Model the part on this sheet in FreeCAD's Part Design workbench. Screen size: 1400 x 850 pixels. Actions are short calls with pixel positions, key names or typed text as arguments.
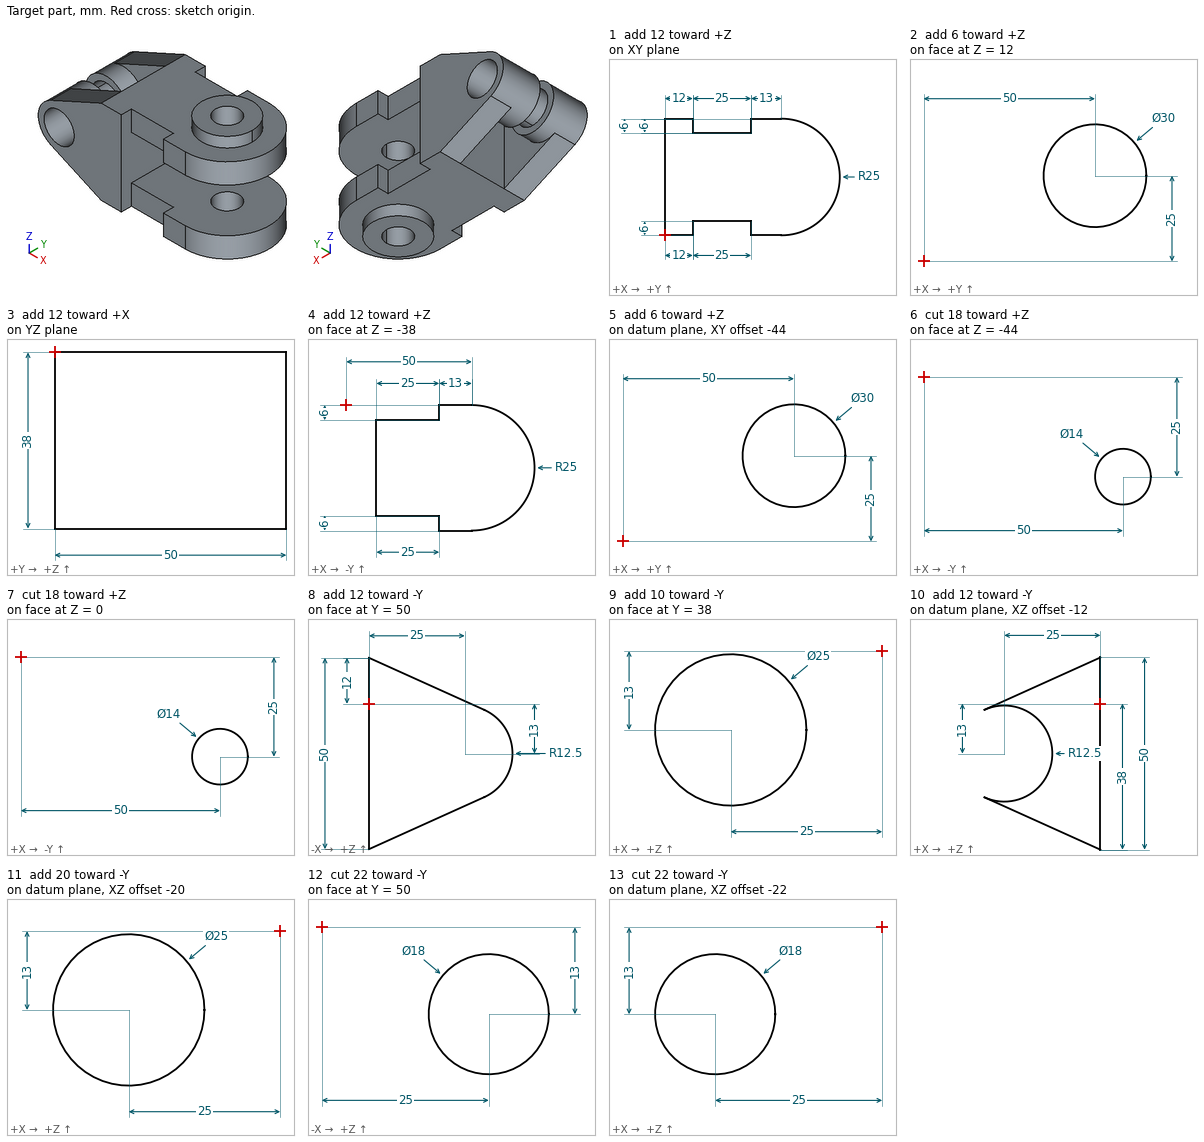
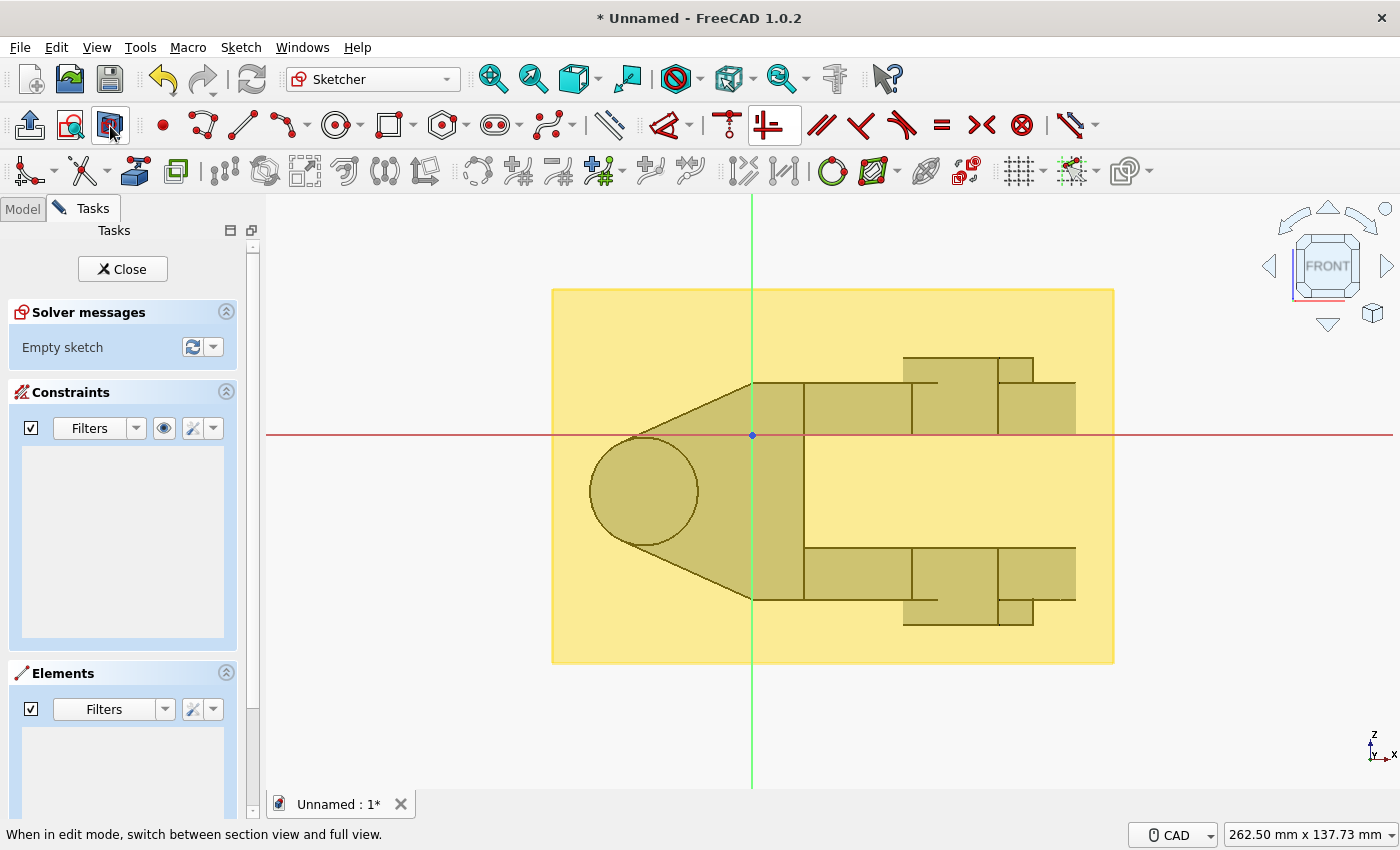
scroll(592, 491, up, 3)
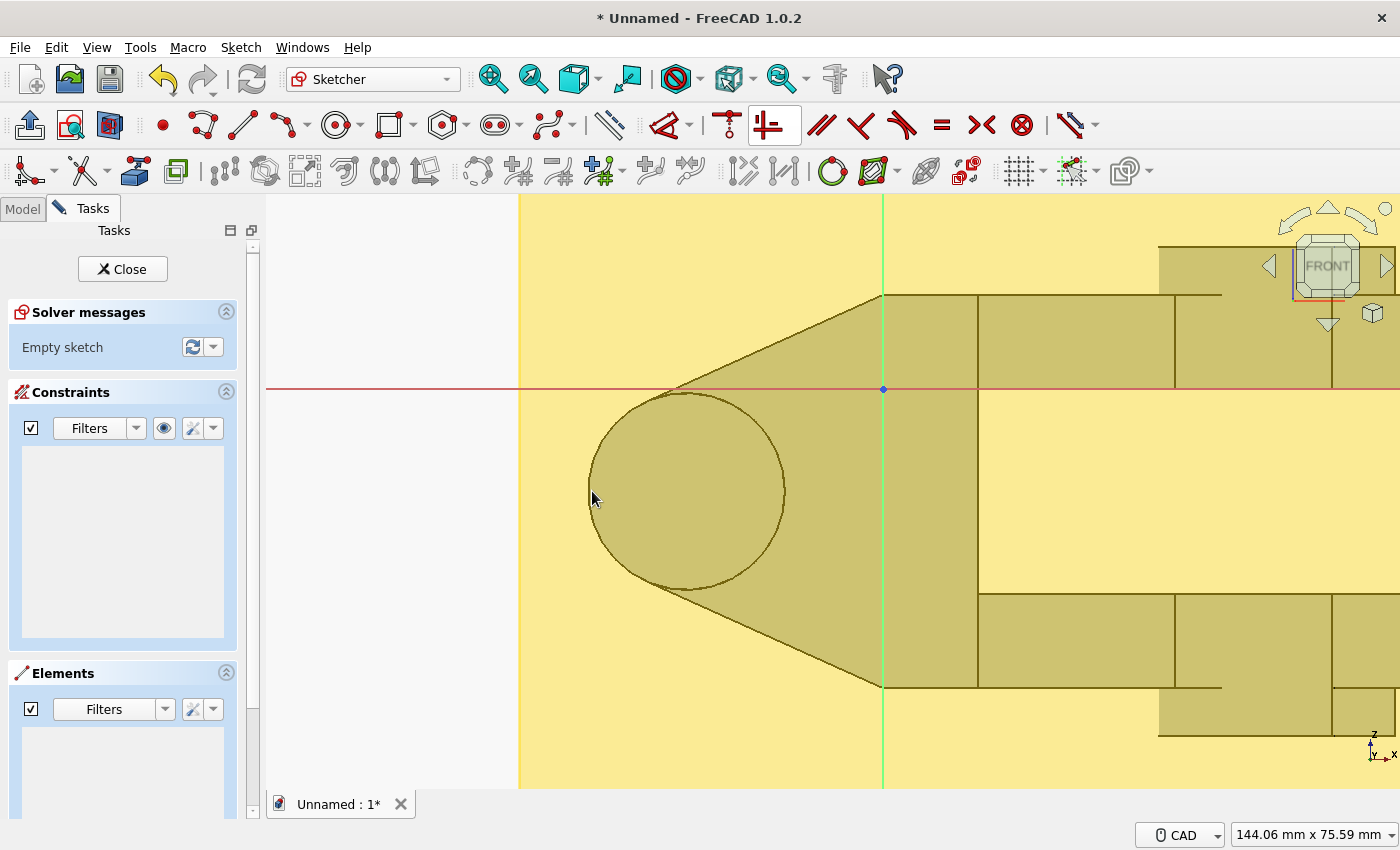
click(204, 126)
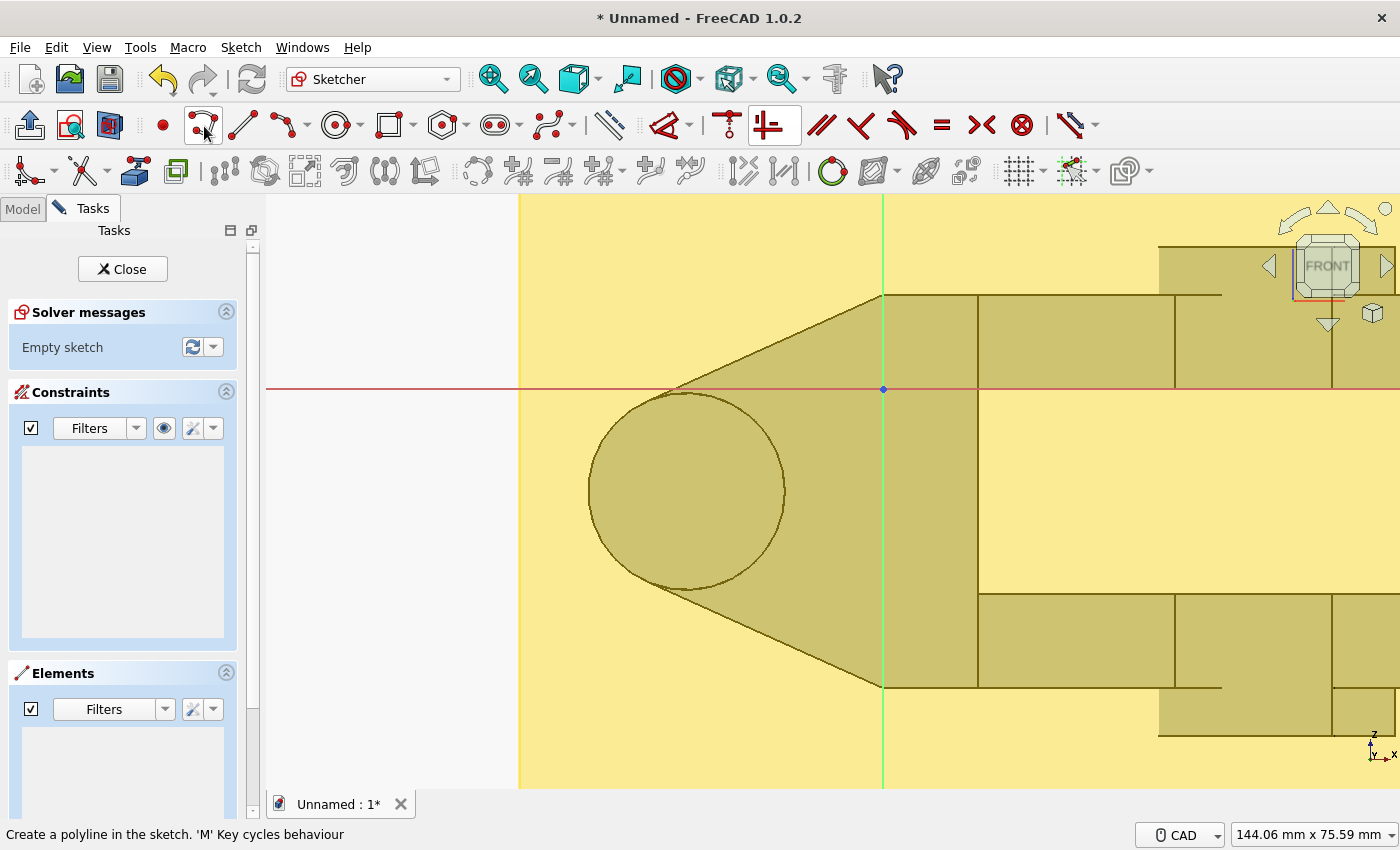
click(646, 581)
click(883, 688)
click(874, 295)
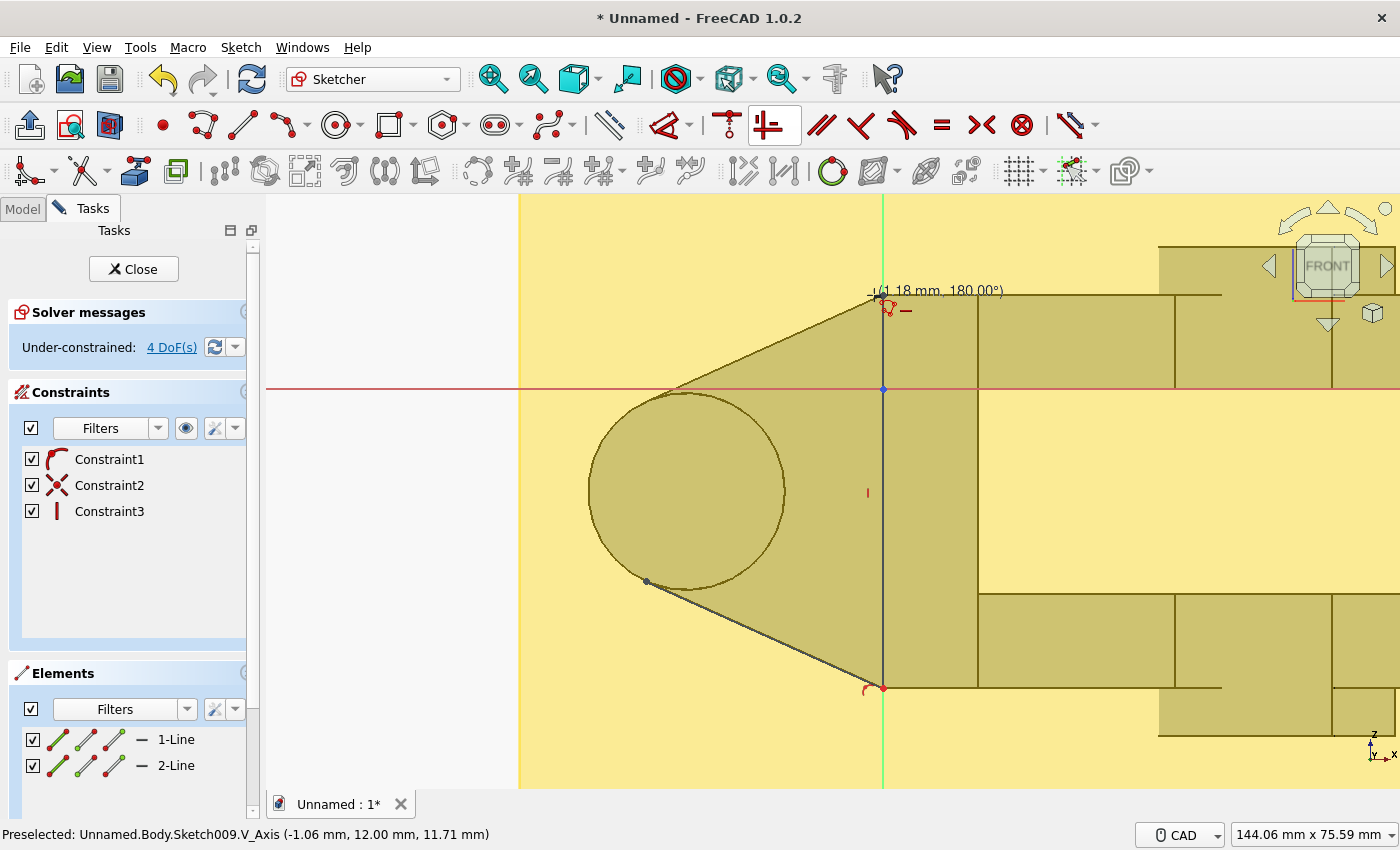
scroll(646, 402, up, 2)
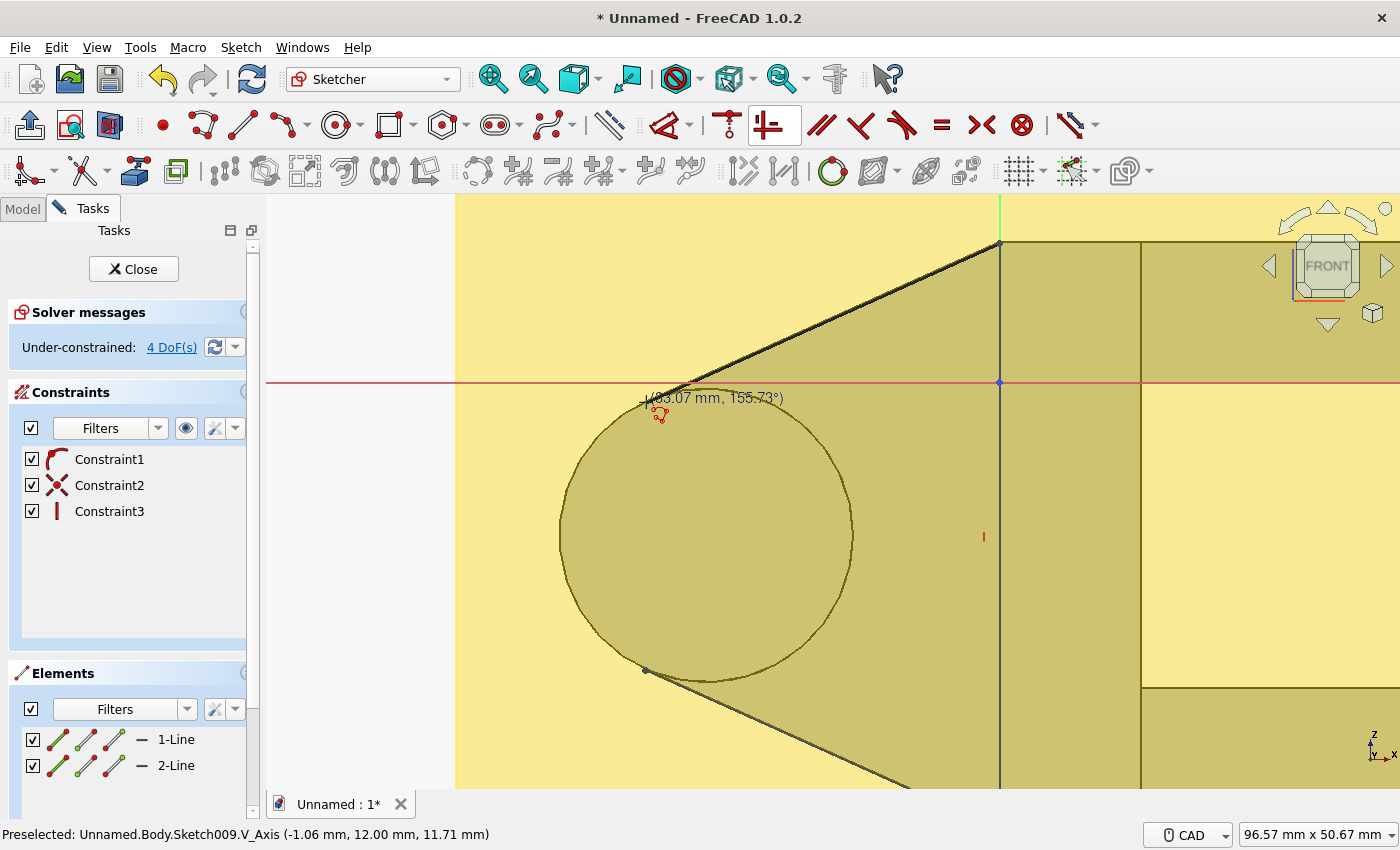
click(646, 402)
right_click(646, 402)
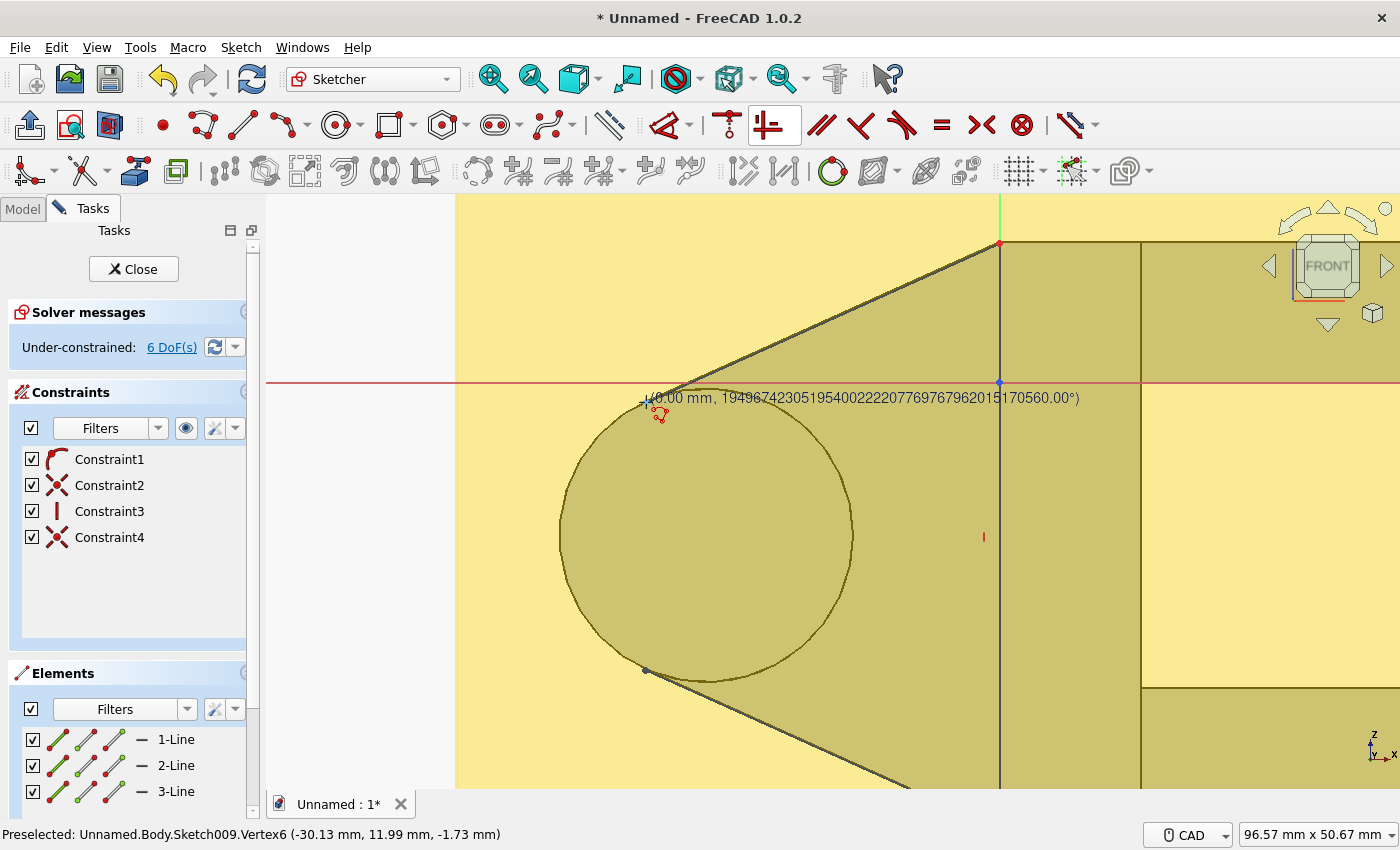
key(g)
key(3)
key(a)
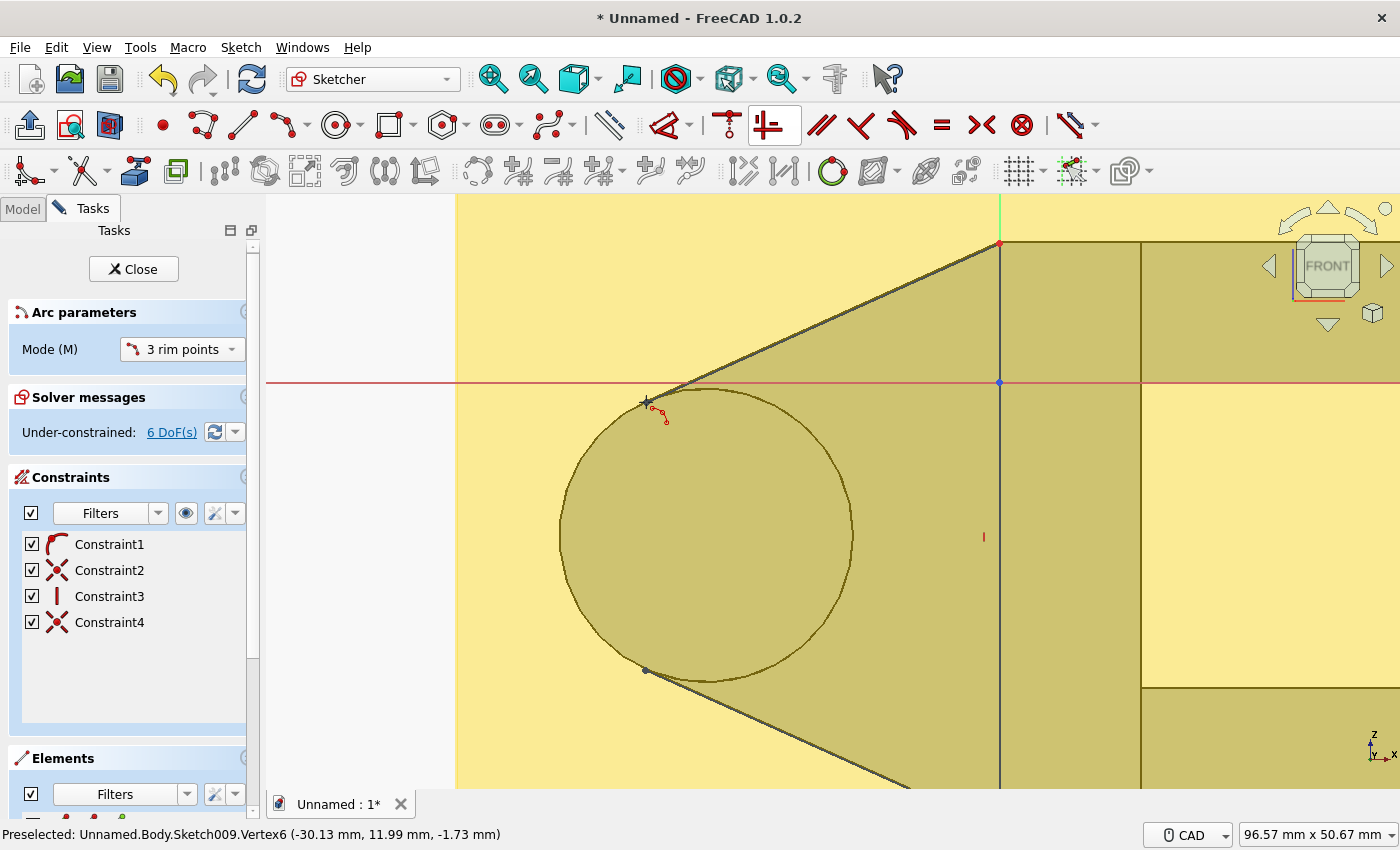
click(646, 403)
click(646, 670)
click(853, 535)
key(Escape)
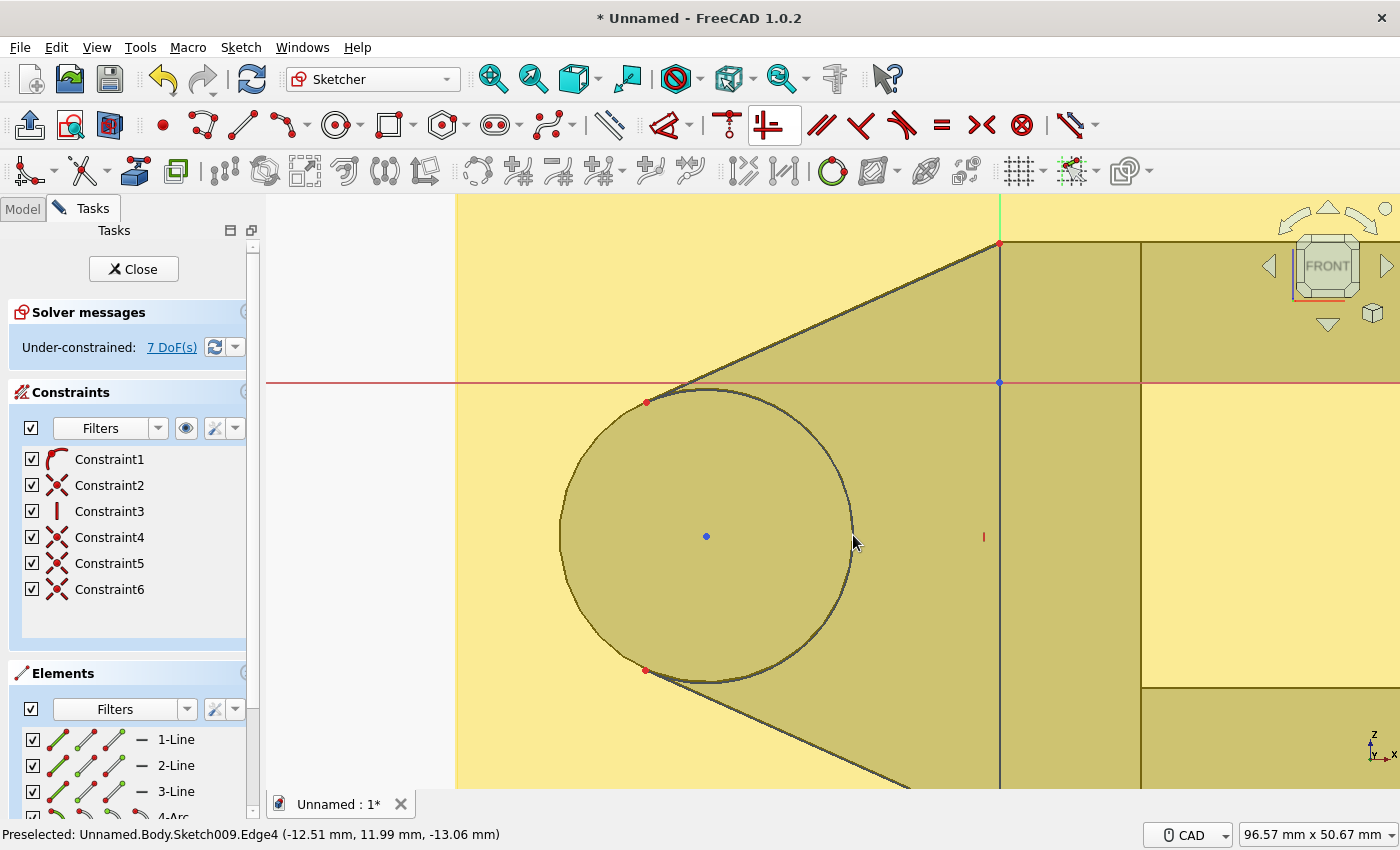
click(752, 718)